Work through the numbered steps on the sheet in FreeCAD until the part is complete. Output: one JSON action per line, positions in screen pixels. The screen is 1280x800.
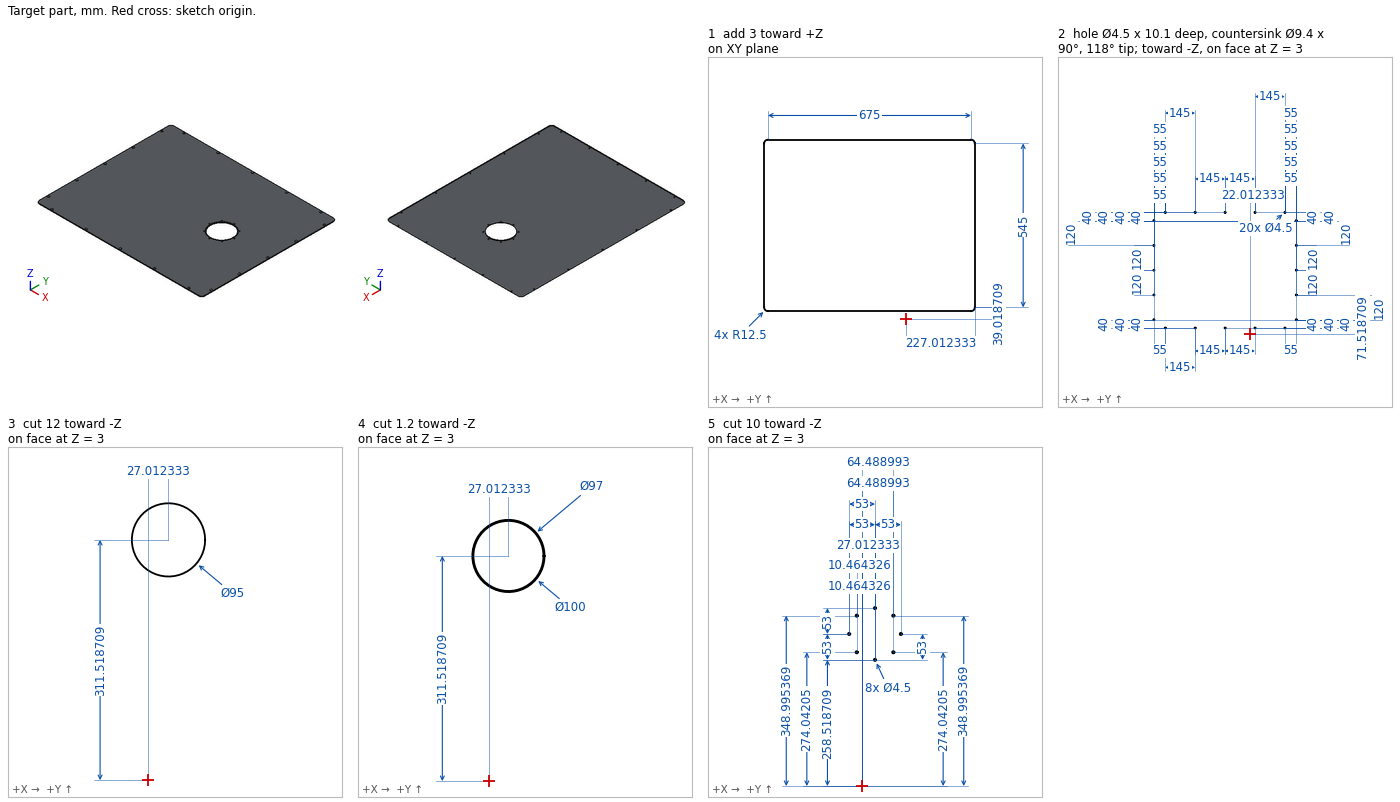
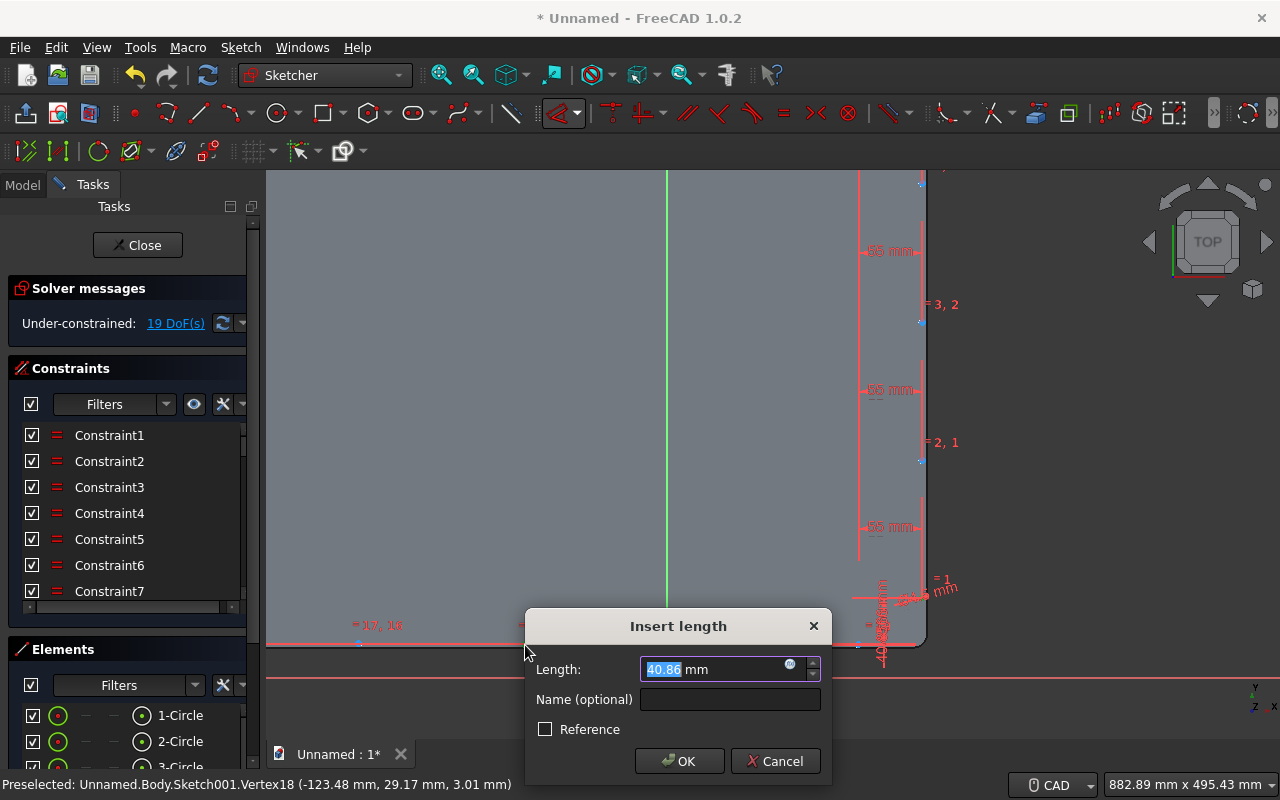
{"action": "type", "text": "40"}
{"action": "key", "text": "Return"}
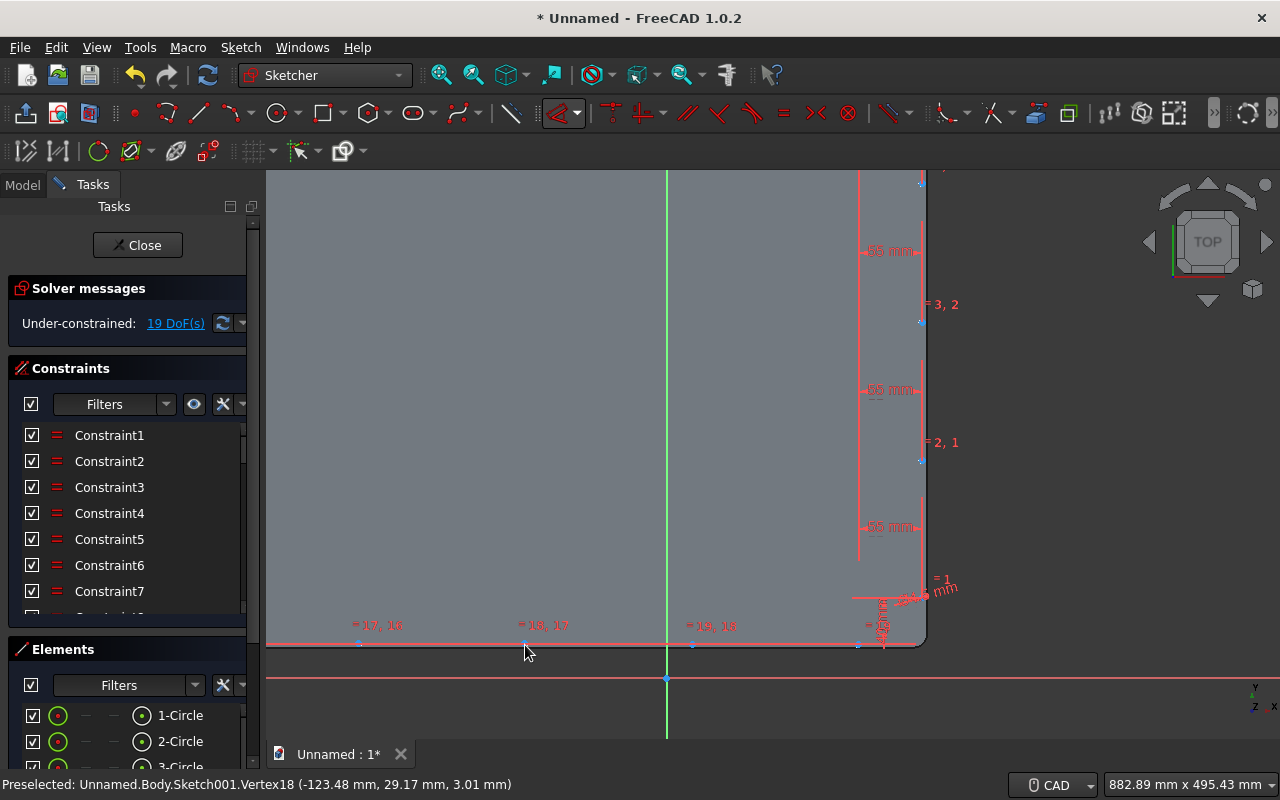
{"action": "left_click", "coordinate": [922, 598]}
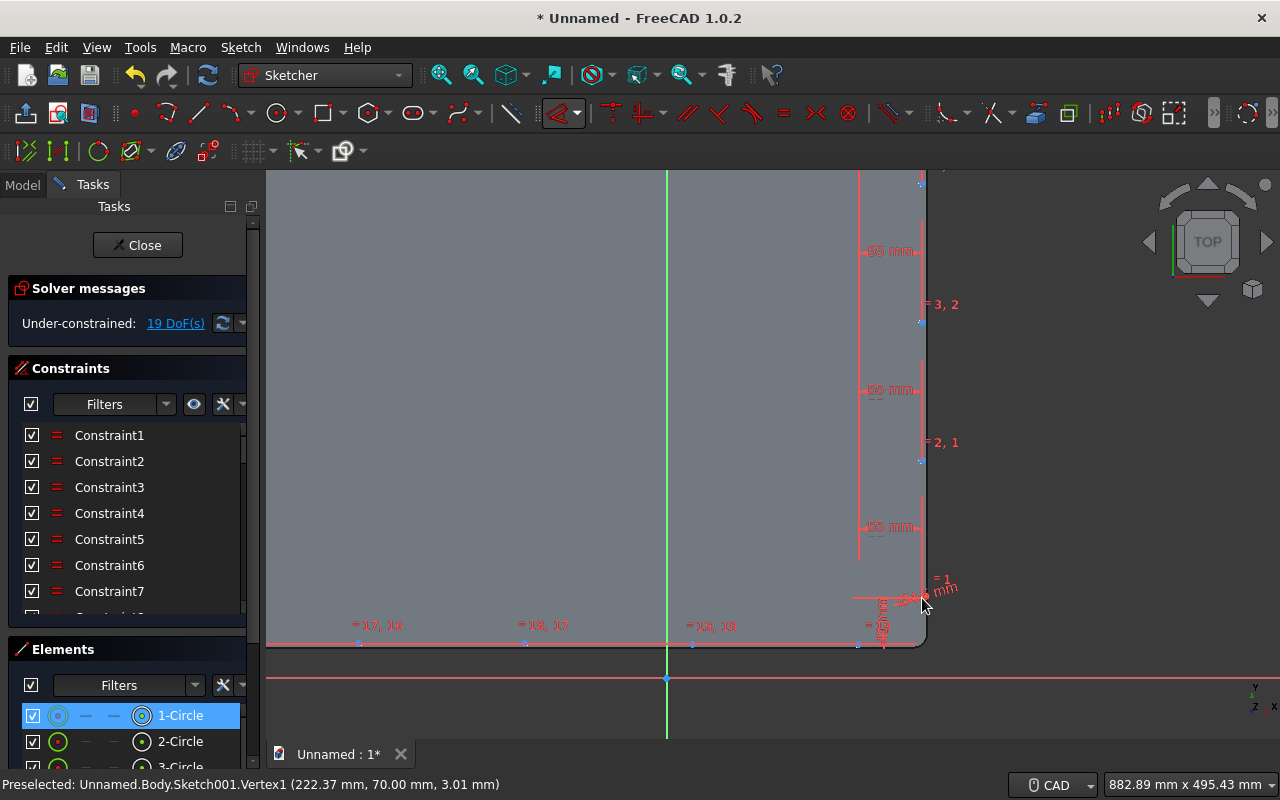
{"action": "left_click", "coordinate": [693, 645]}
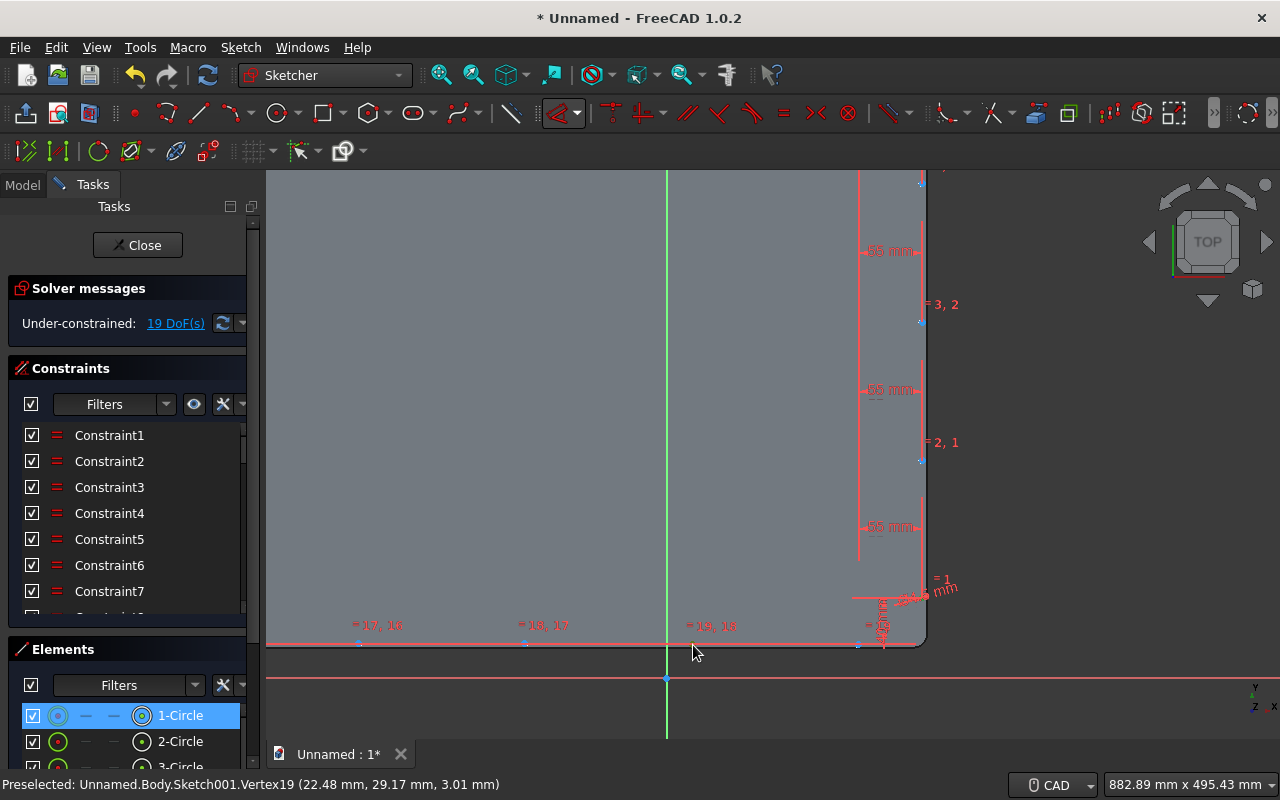
{"action": "key", "text": "i"}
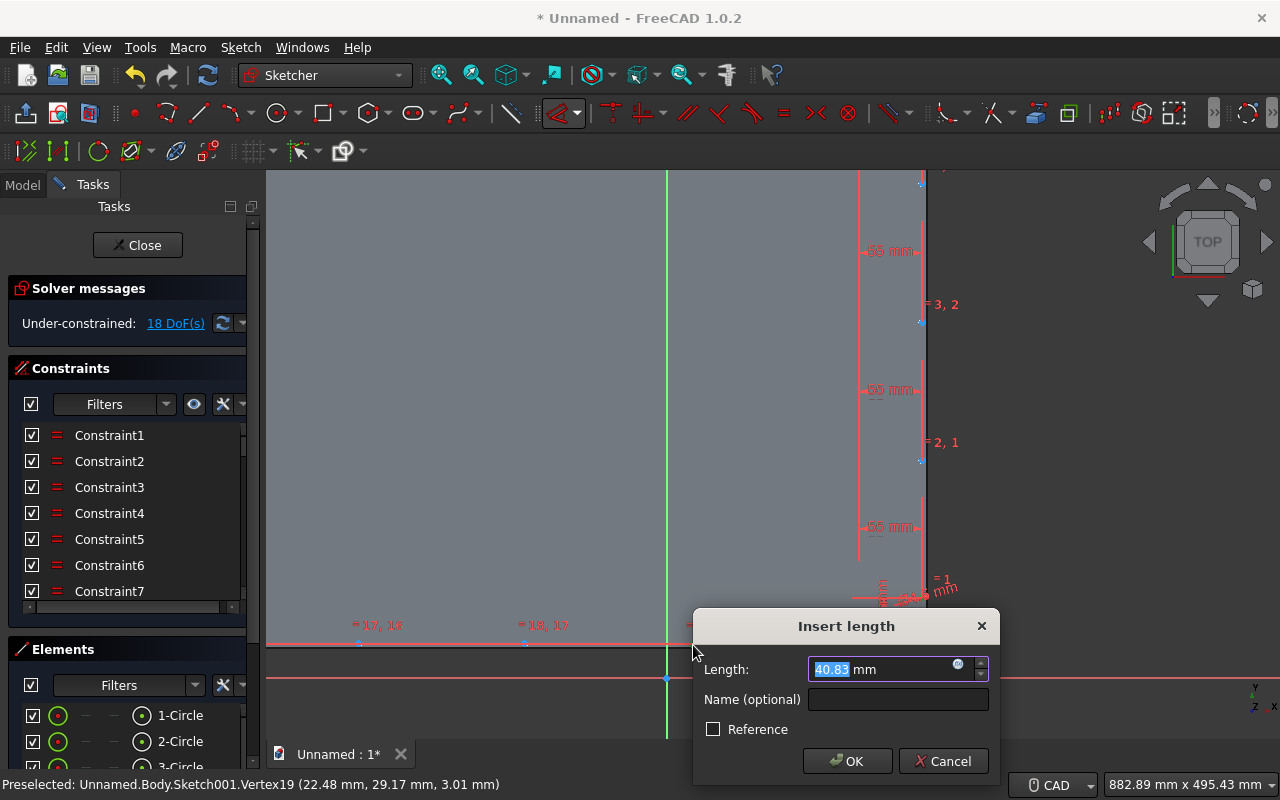
{"action": "type", "text": "40"}
{"action": "key", "text": "Return"}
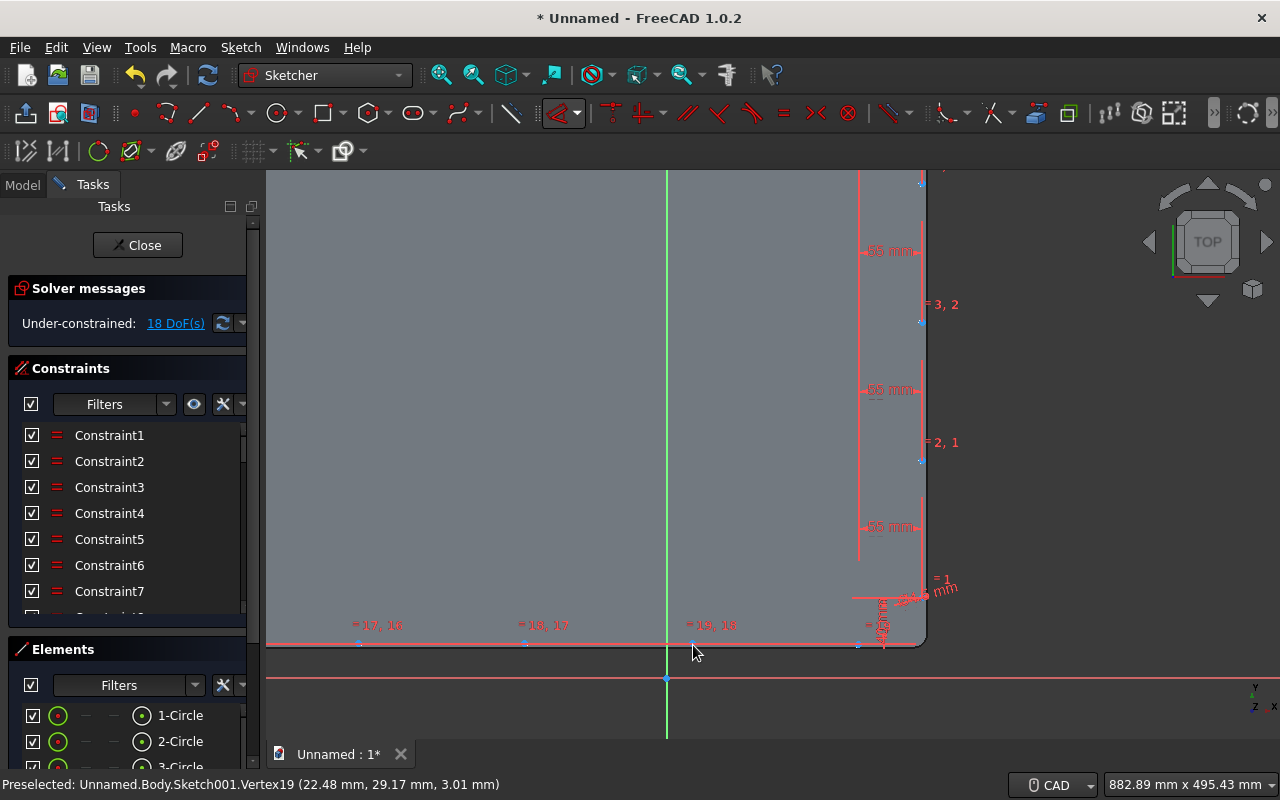
{"action": "left_click", "coordinate": [922, 598]}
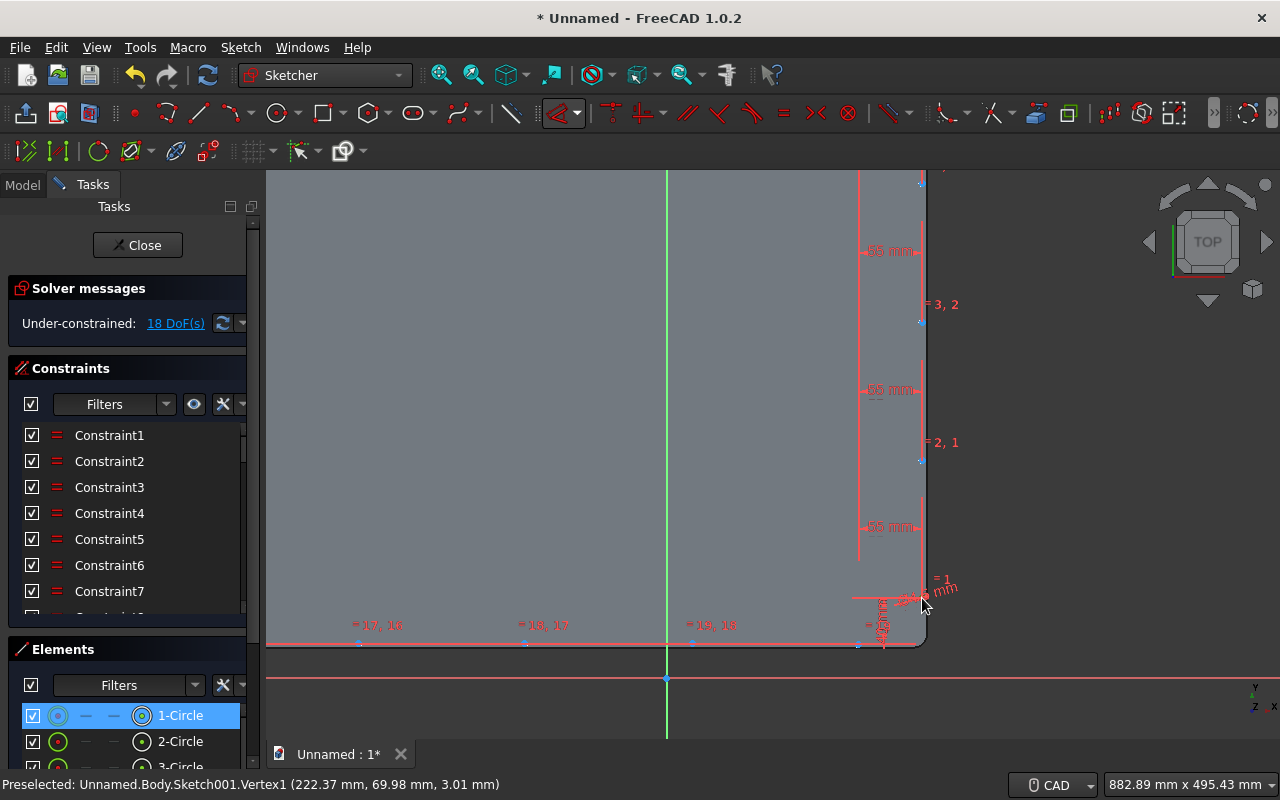
{"action": "left_click", "coordinate": [858, 645]}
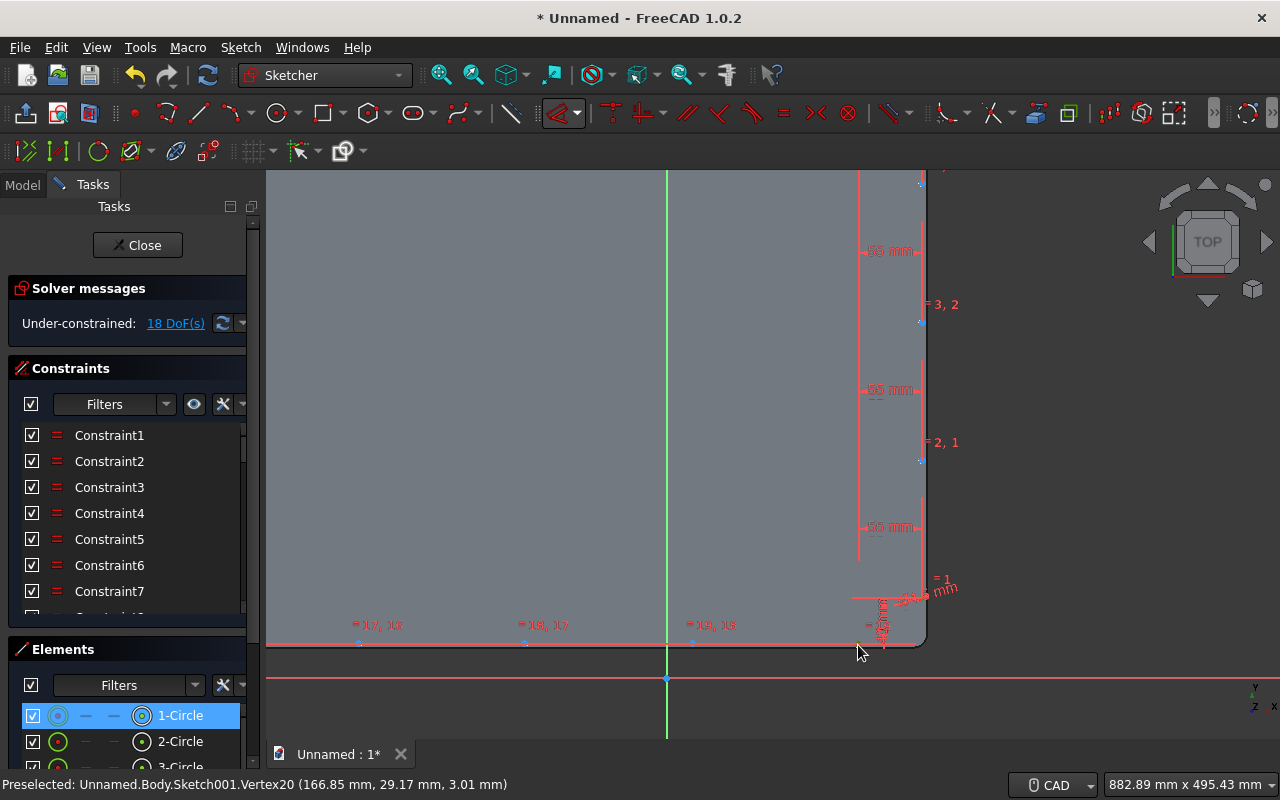
{"action": "left_click", "coordinate": [580, 114]}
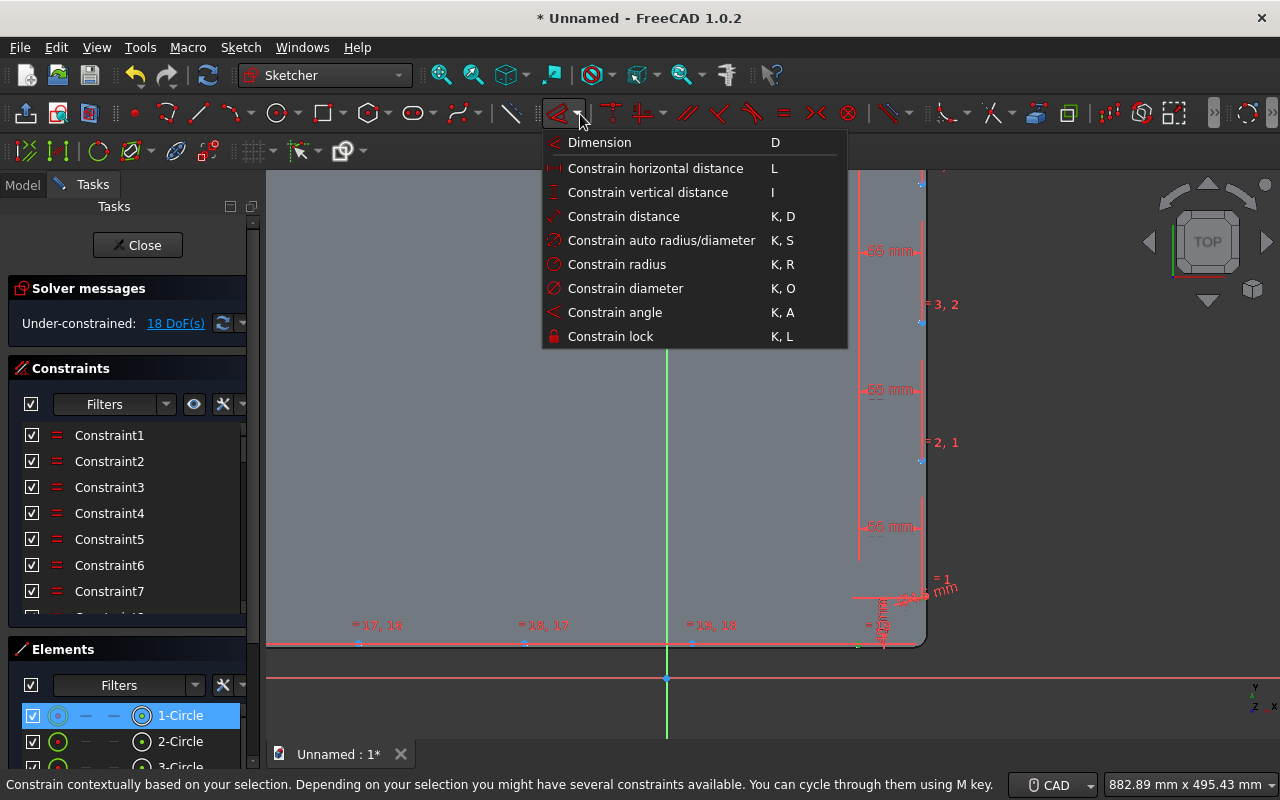
{"action": "left_click", "coordinate": [695, 168]}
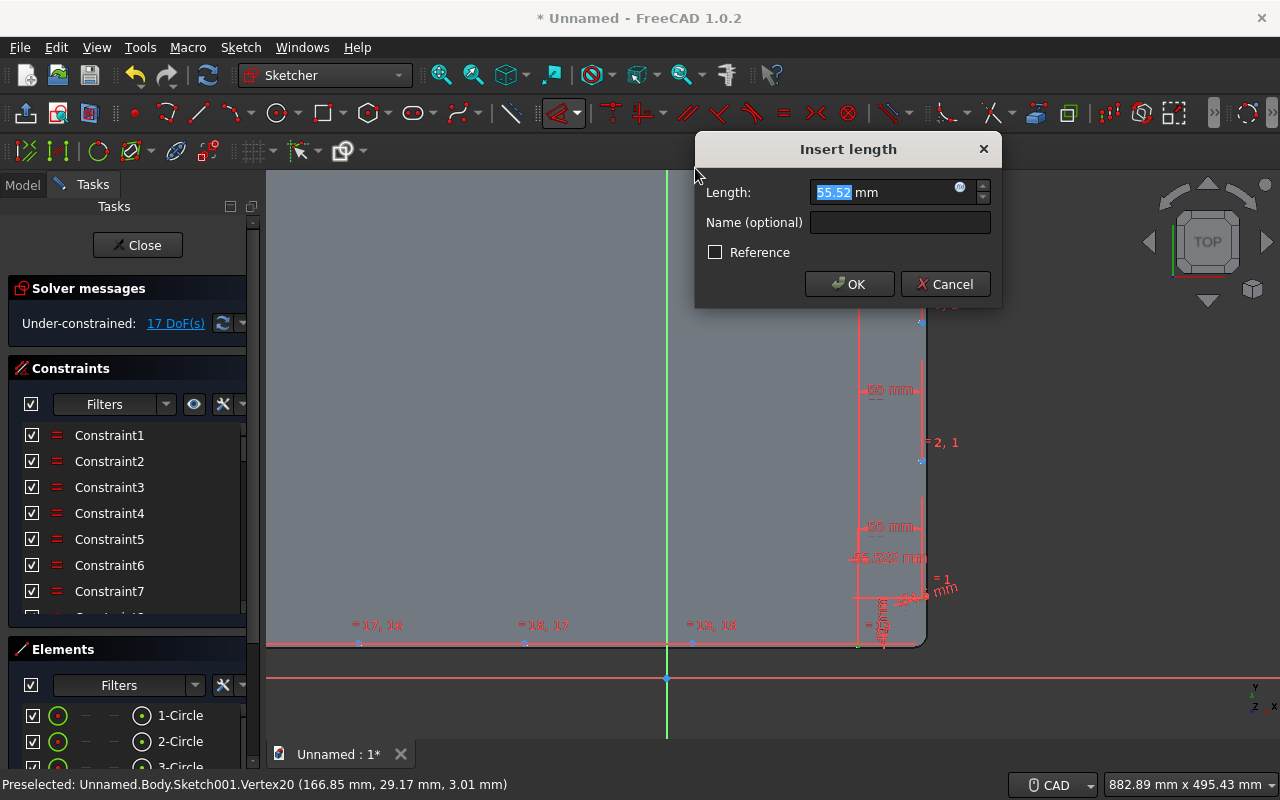
{"action": "type", "text": "55"}
{"action": "key", "text": "Return"}